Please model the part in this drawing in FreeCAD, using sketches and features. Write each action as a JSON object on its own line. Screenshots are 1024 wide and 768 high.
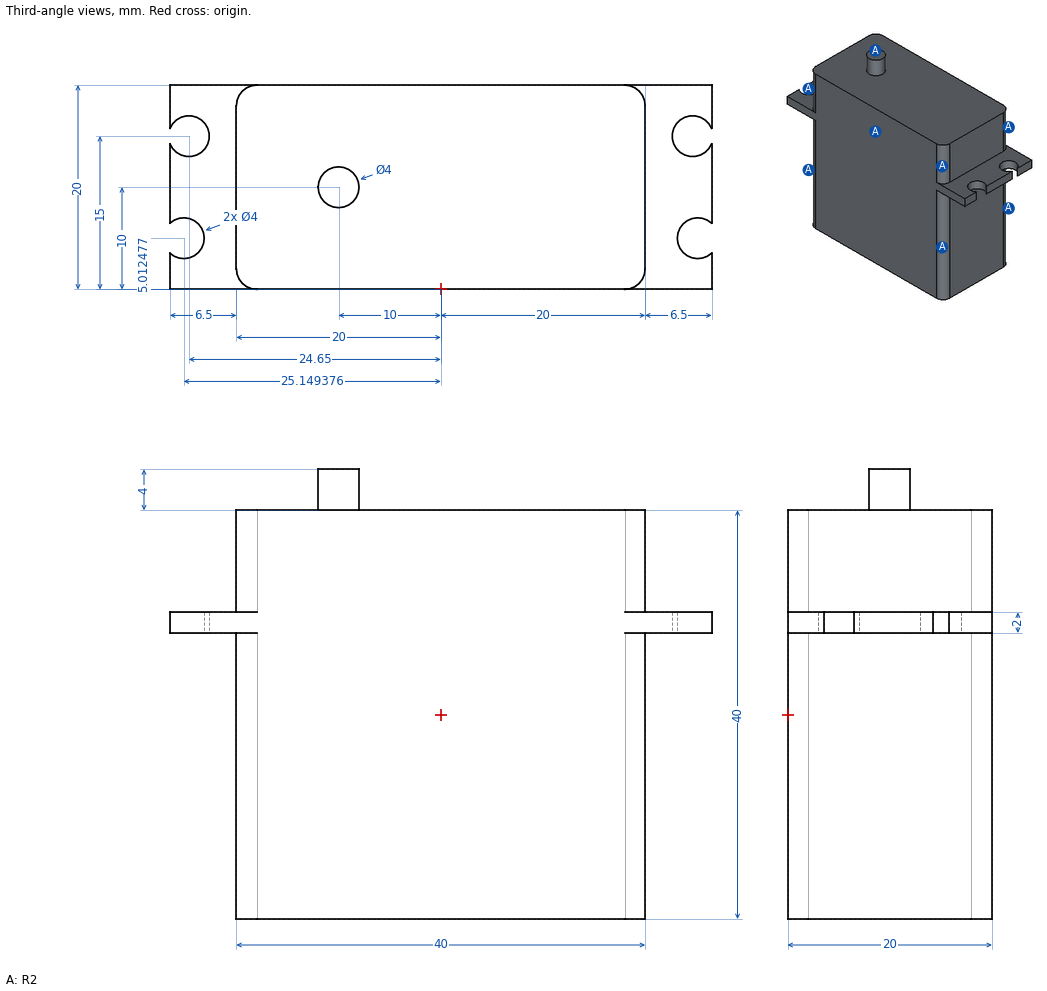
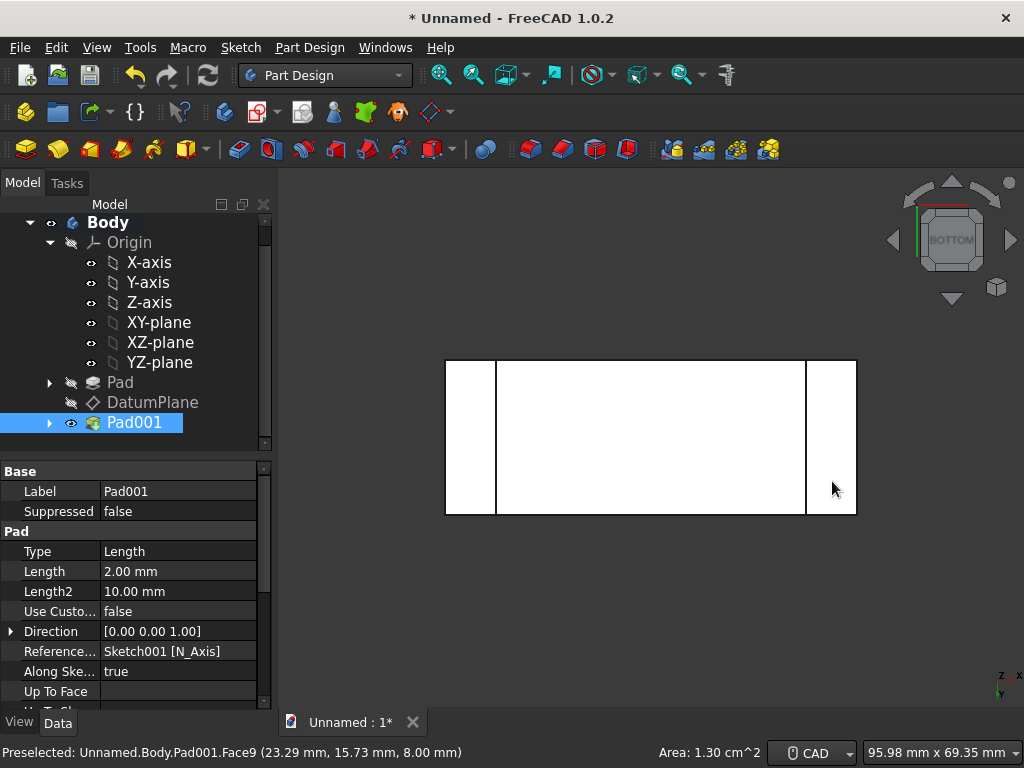
{"action": "left_click", "coordinate": [258, 112]}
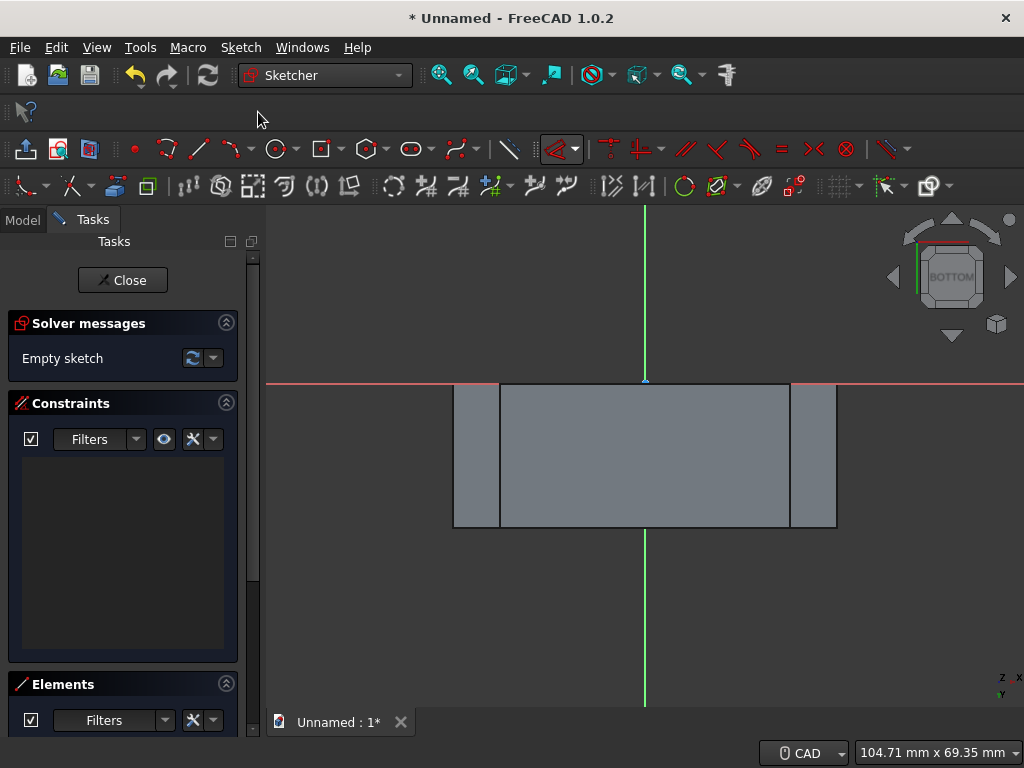
{"action": "scroll", "coordinate": [522, 436], "scroll_direction": "up", "scroll_amount": 4}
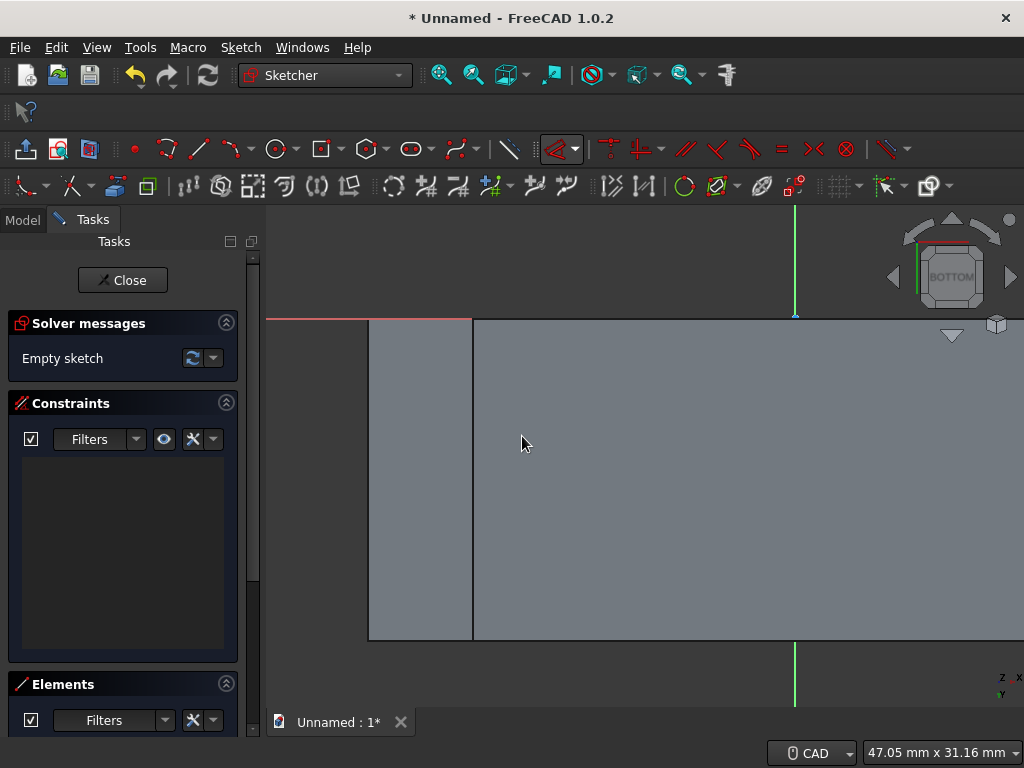
{"action": "key", "text": "g c"}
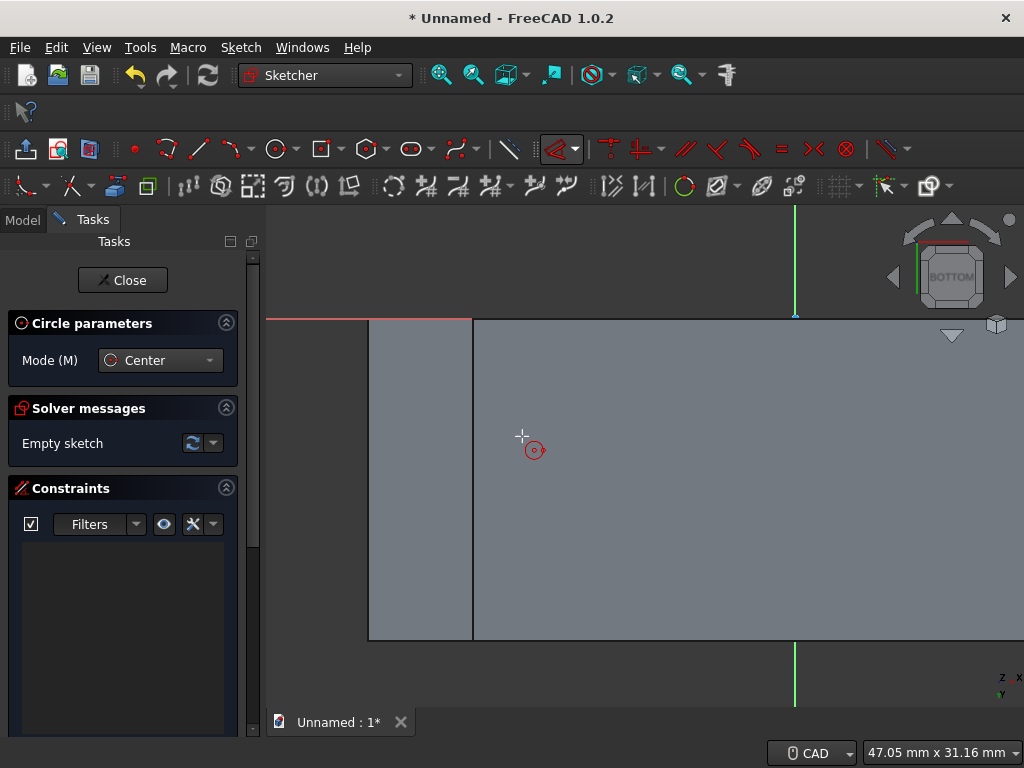
{"action": "left_click", "coordinate": [390, 400]}
{"action": "left_click", "coordinate": [413, 377]}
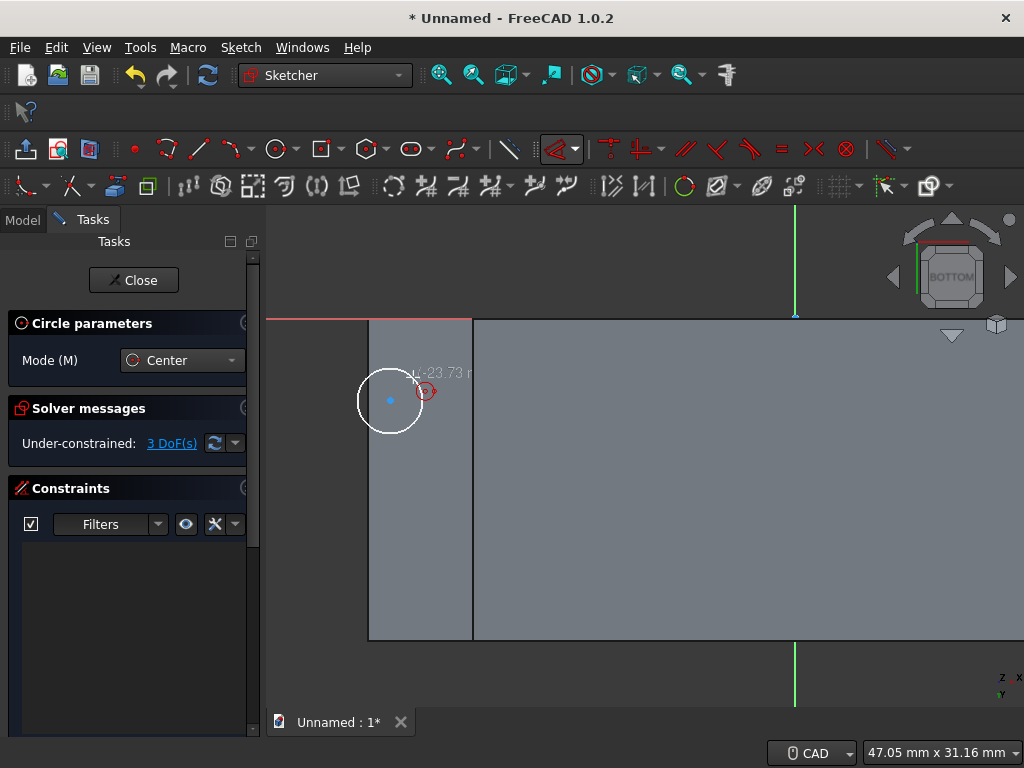
{"action": "left_click", "coordinate": [398, 560]}
{"action": "left_click", "coordinate": [421, 538]}
{"action": "key", "text": "Escape"}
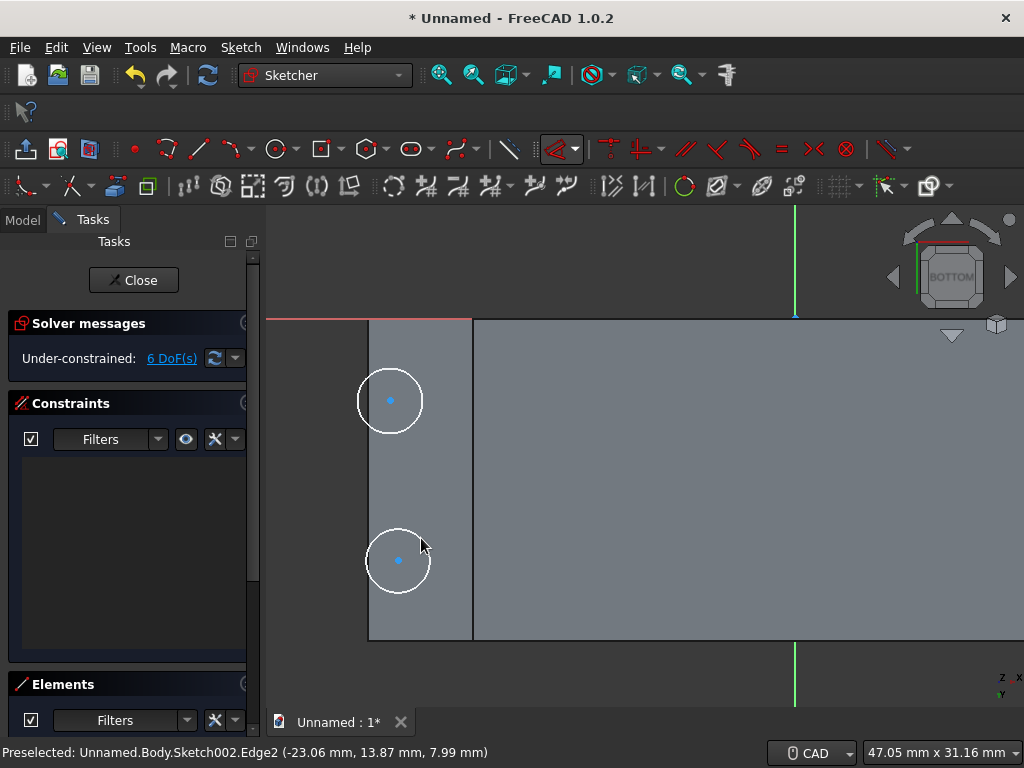
{"action": "left_click", "coordinate": [413, 378]}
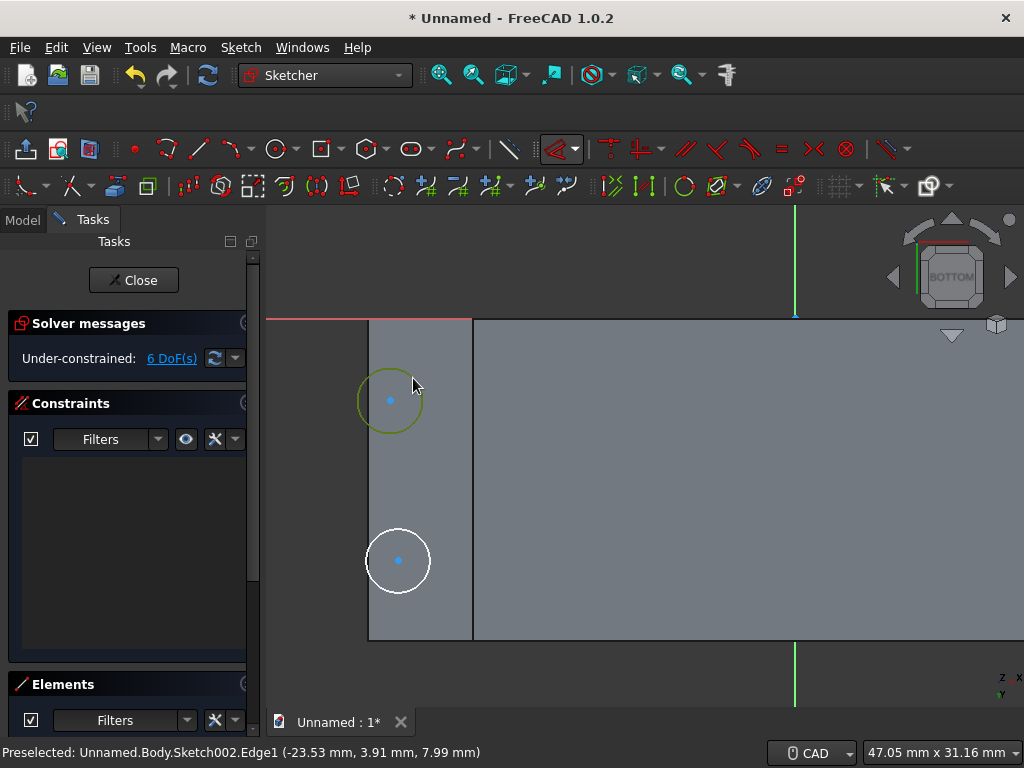
{"action": "left_click", "coordinate": [420, 538]}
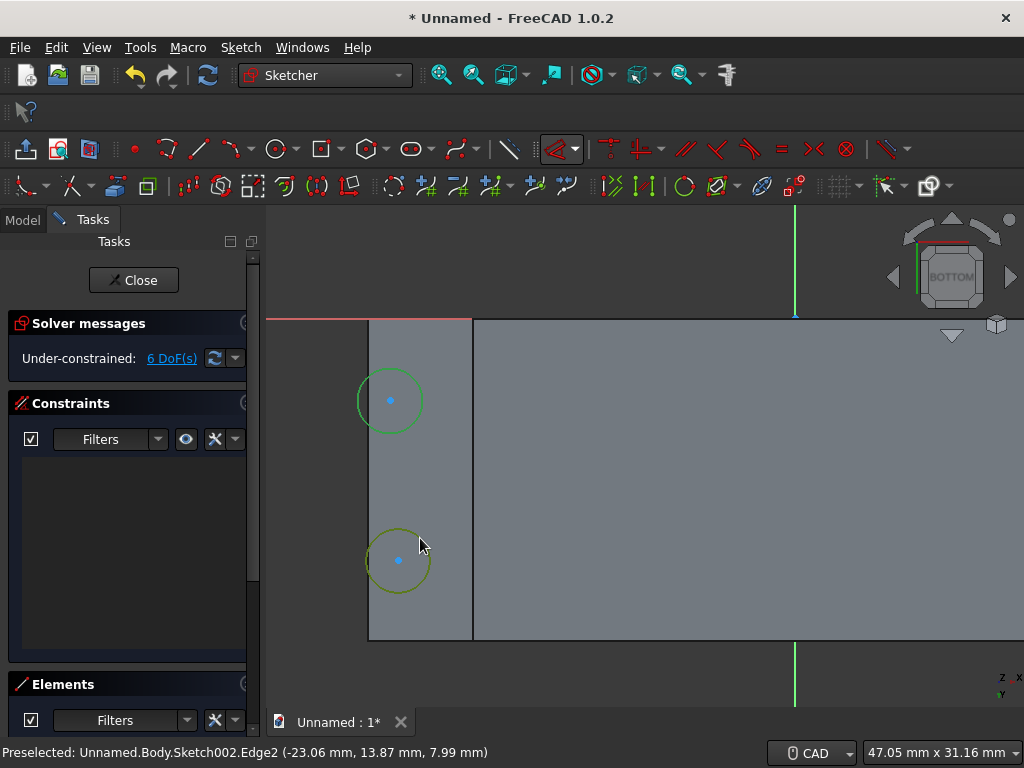
{"action": "key", "text": "e"}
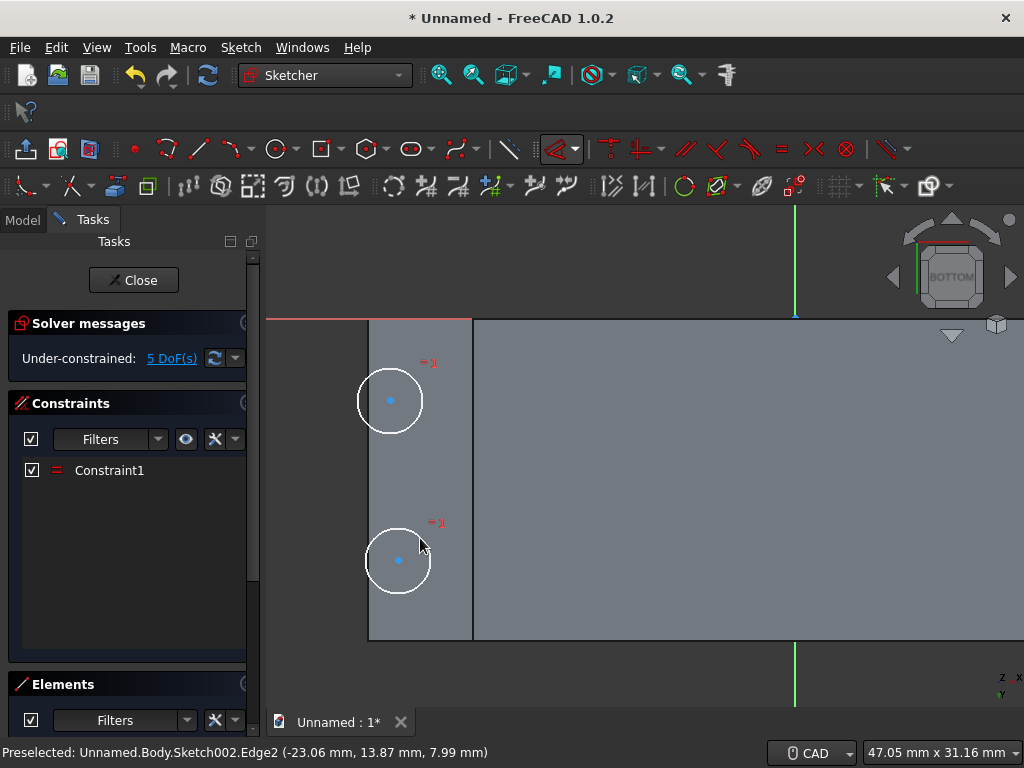
{"action": "left_click", "coordinate": [413, 378]}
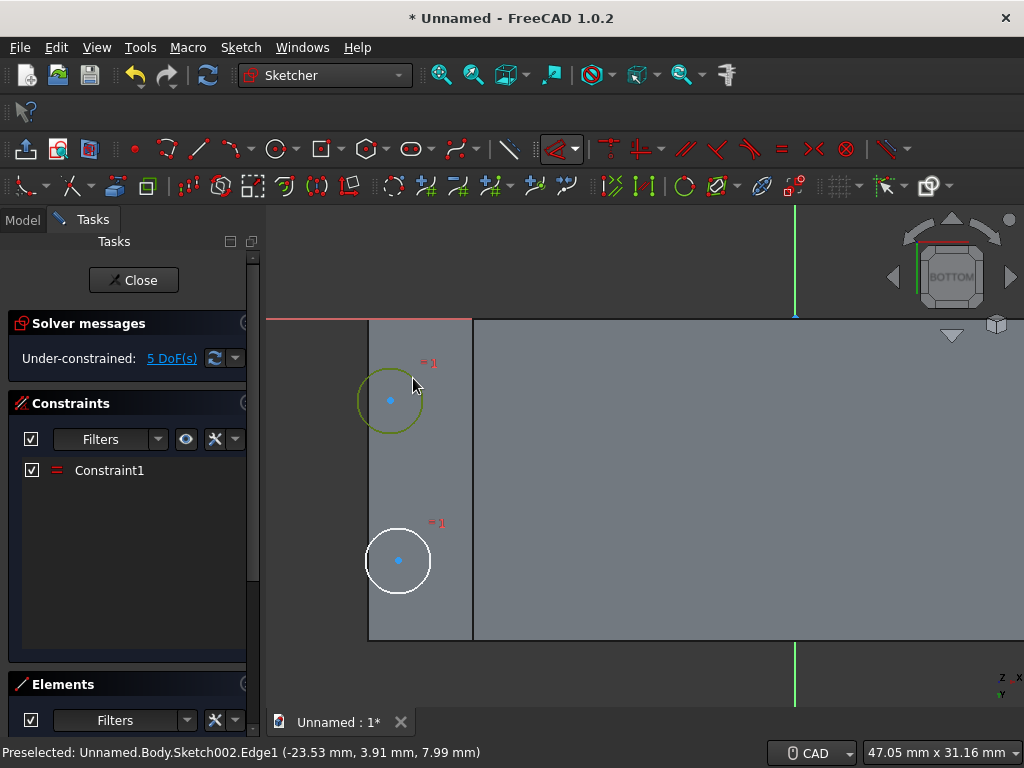
{"action": "left_click", "coordinate": [578, 150]}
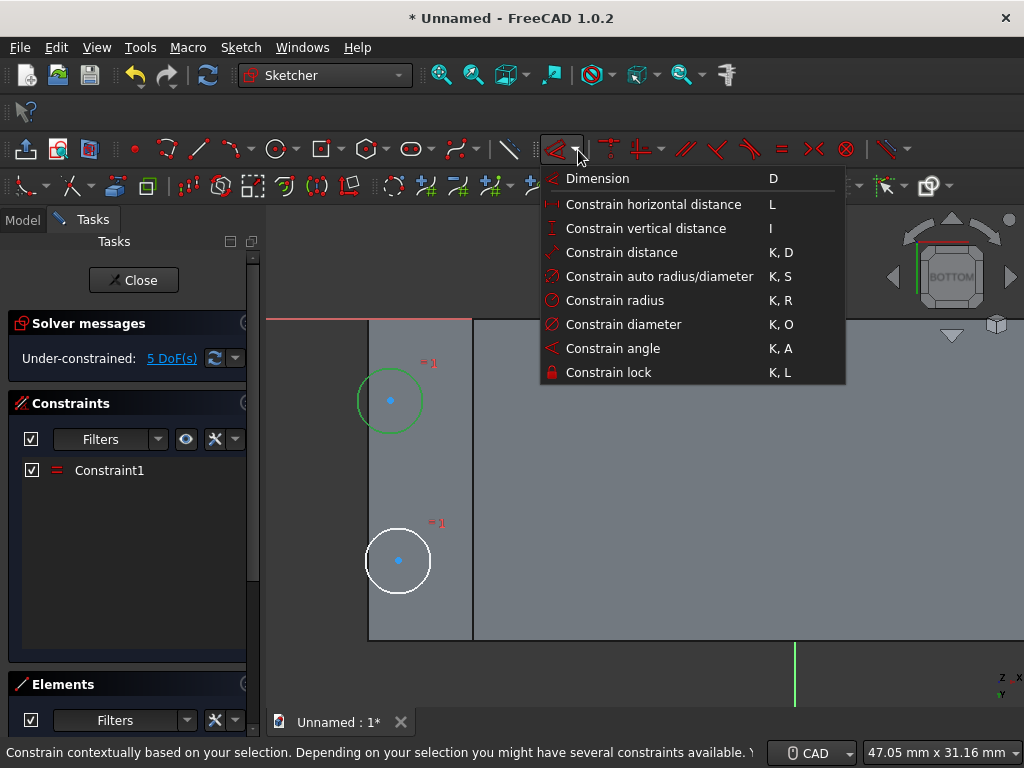
{"action": "left_click", "coordinate": [693, 324]}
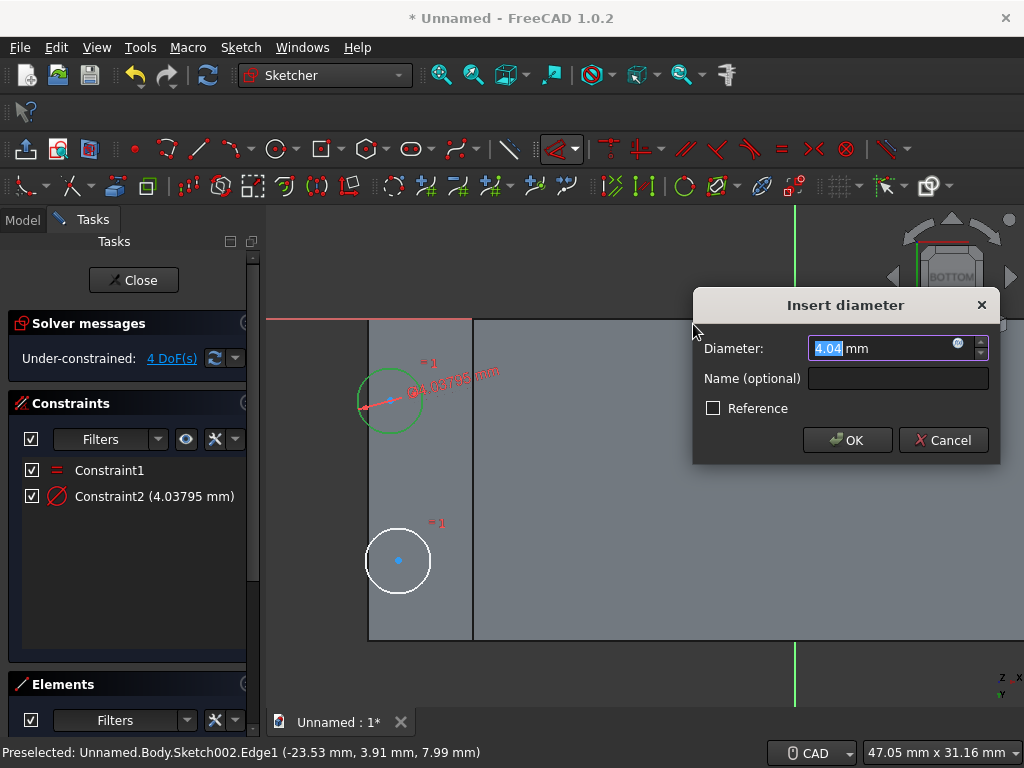
{"action": "type", "text": "4"}
{"action": "key", "text": "Return"}